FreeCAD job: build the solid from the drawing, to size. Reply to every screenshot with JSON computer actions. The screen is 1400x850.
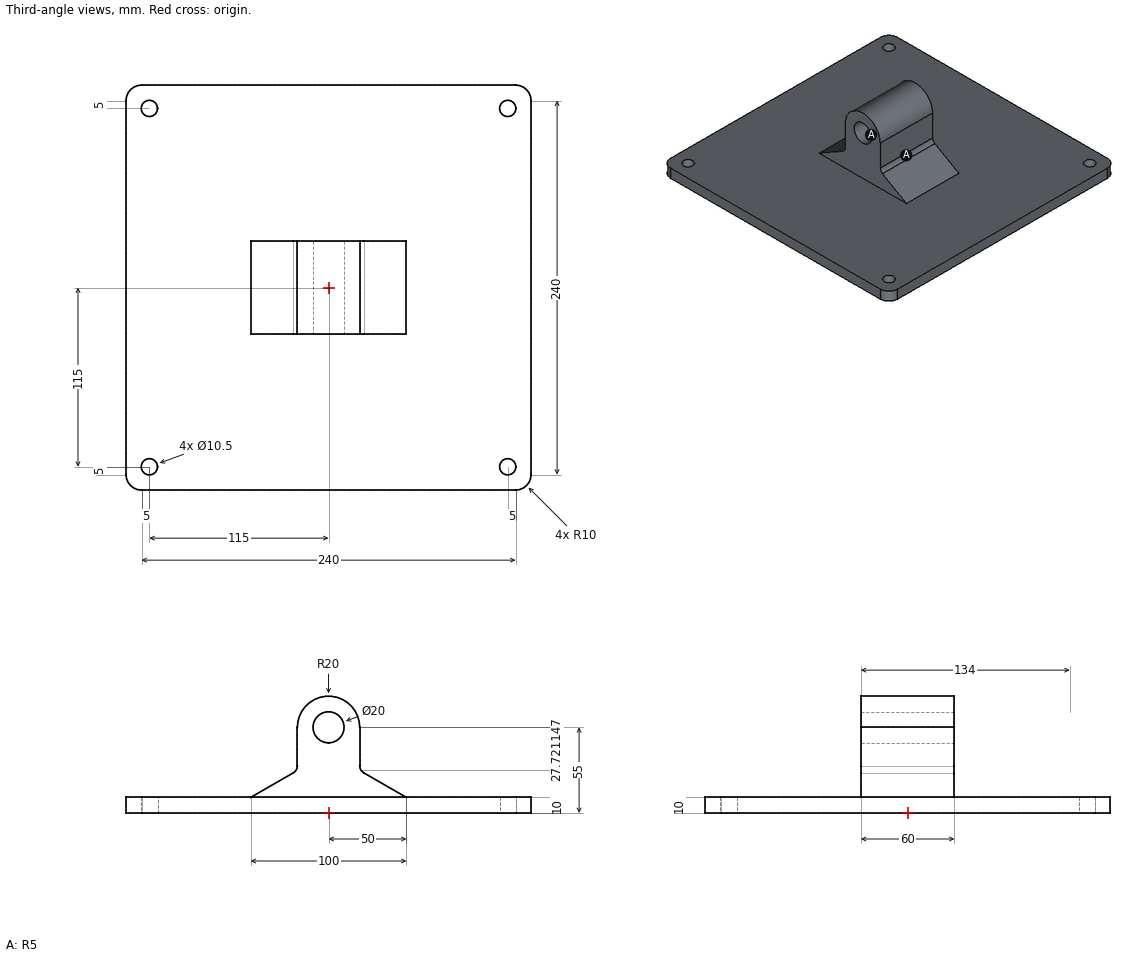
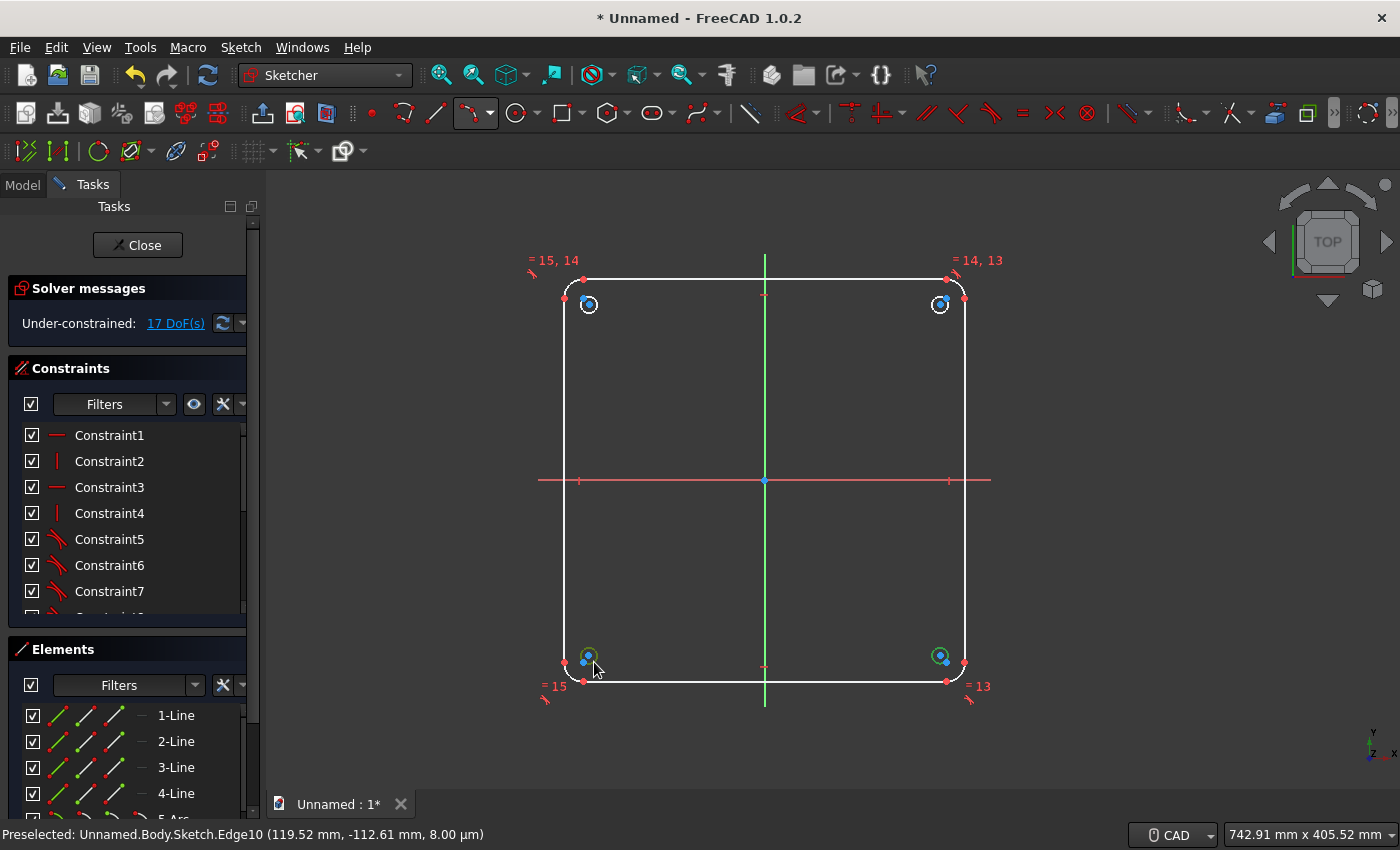
{"action": "scroll", "coordinate": [595, 299], "scroll_direction": "up", "scroll_amount": 3}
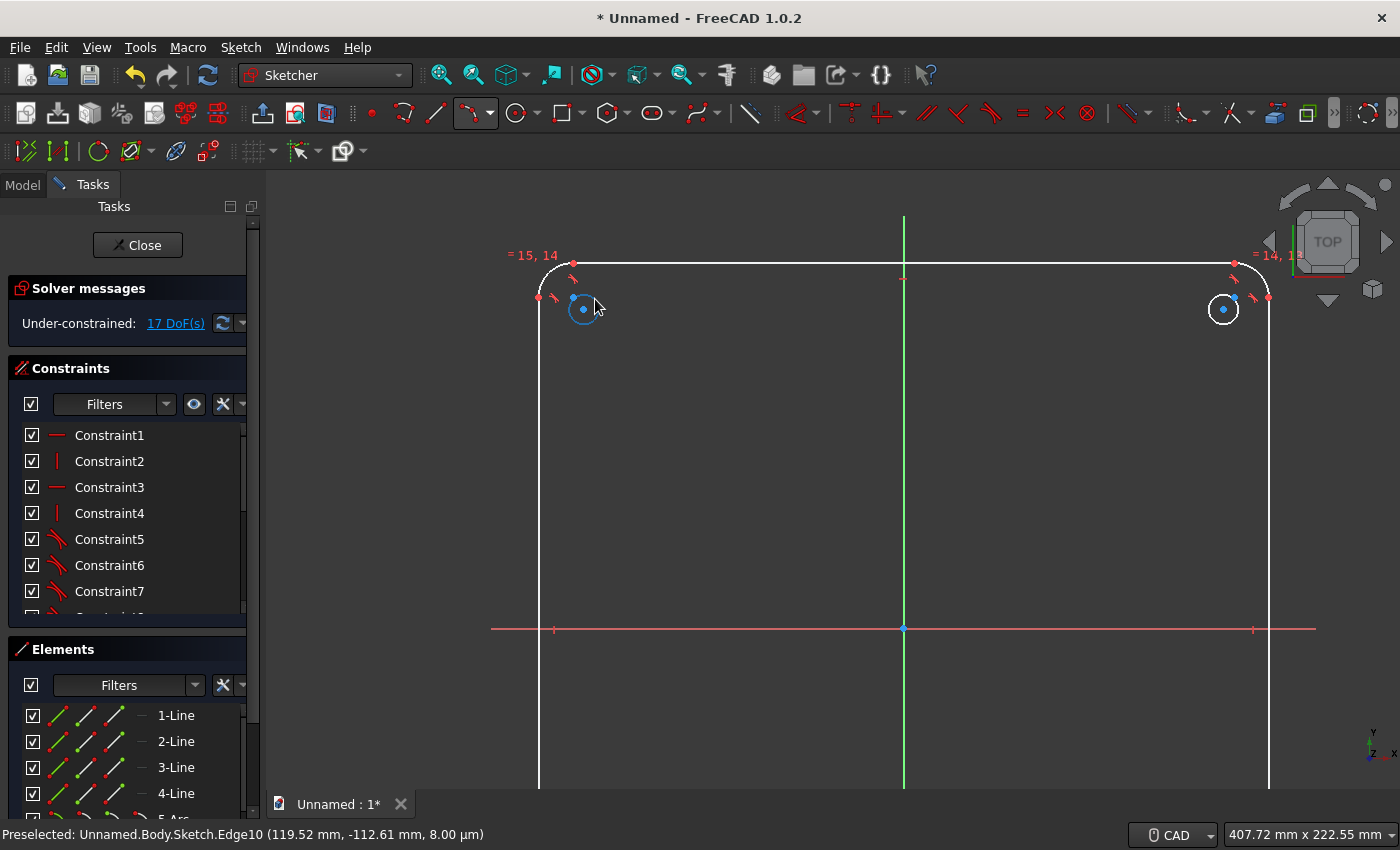
{"action": "left_click", "coordinate": [594, 299]}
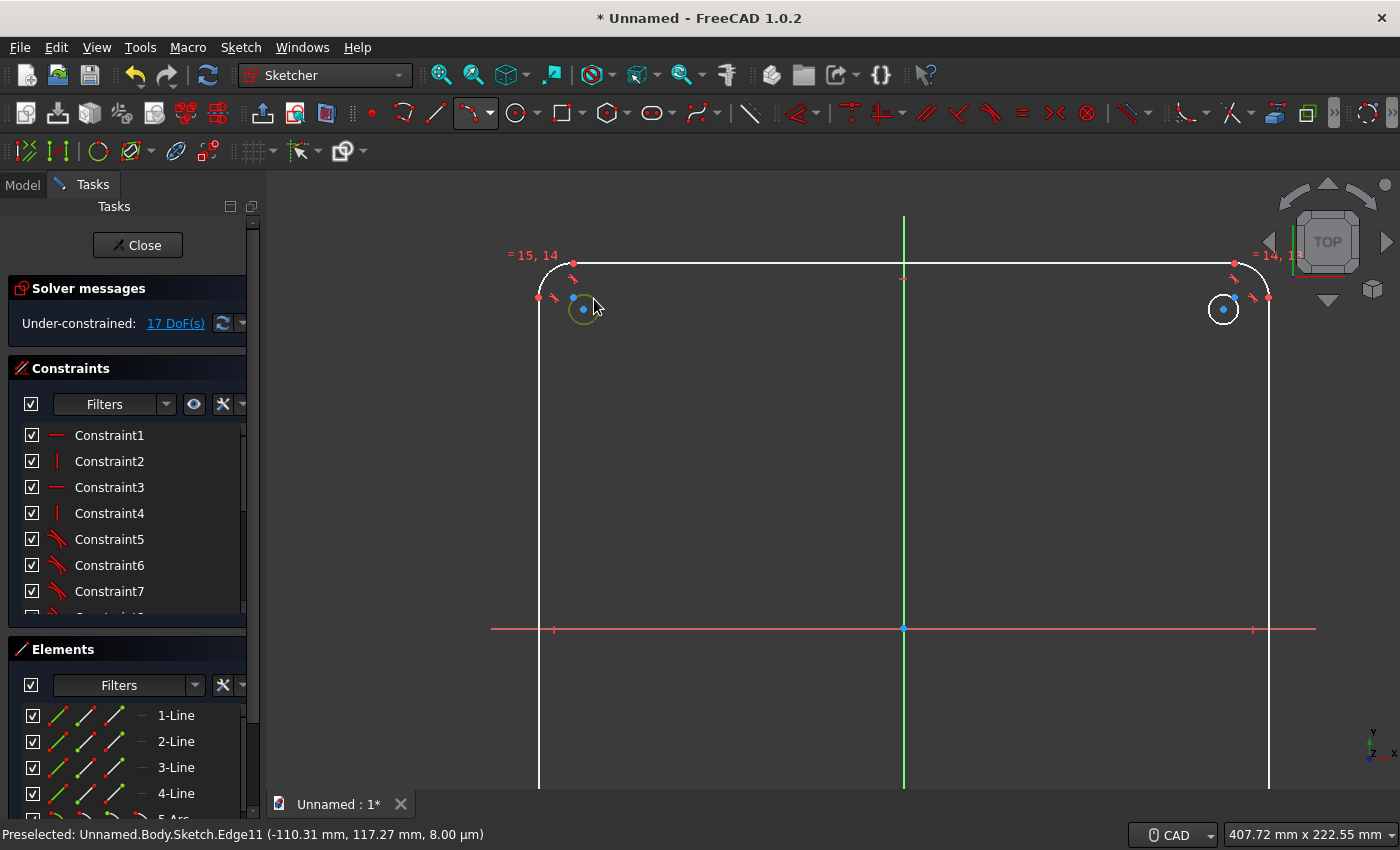
{"action": "left_click", "coordinate": [1213, 299]}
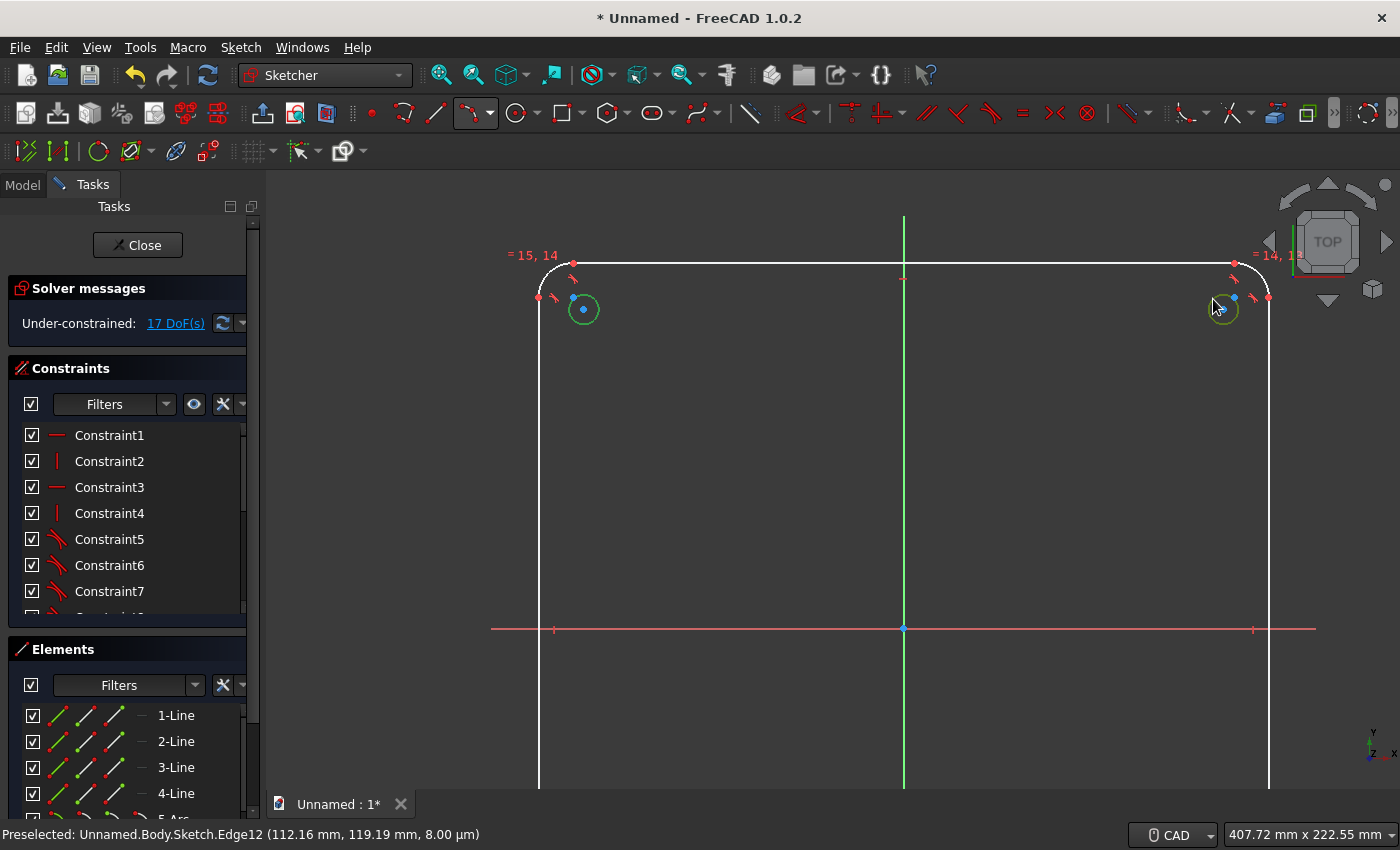
{"action": "left_click", "coordinate": [1024, 114]}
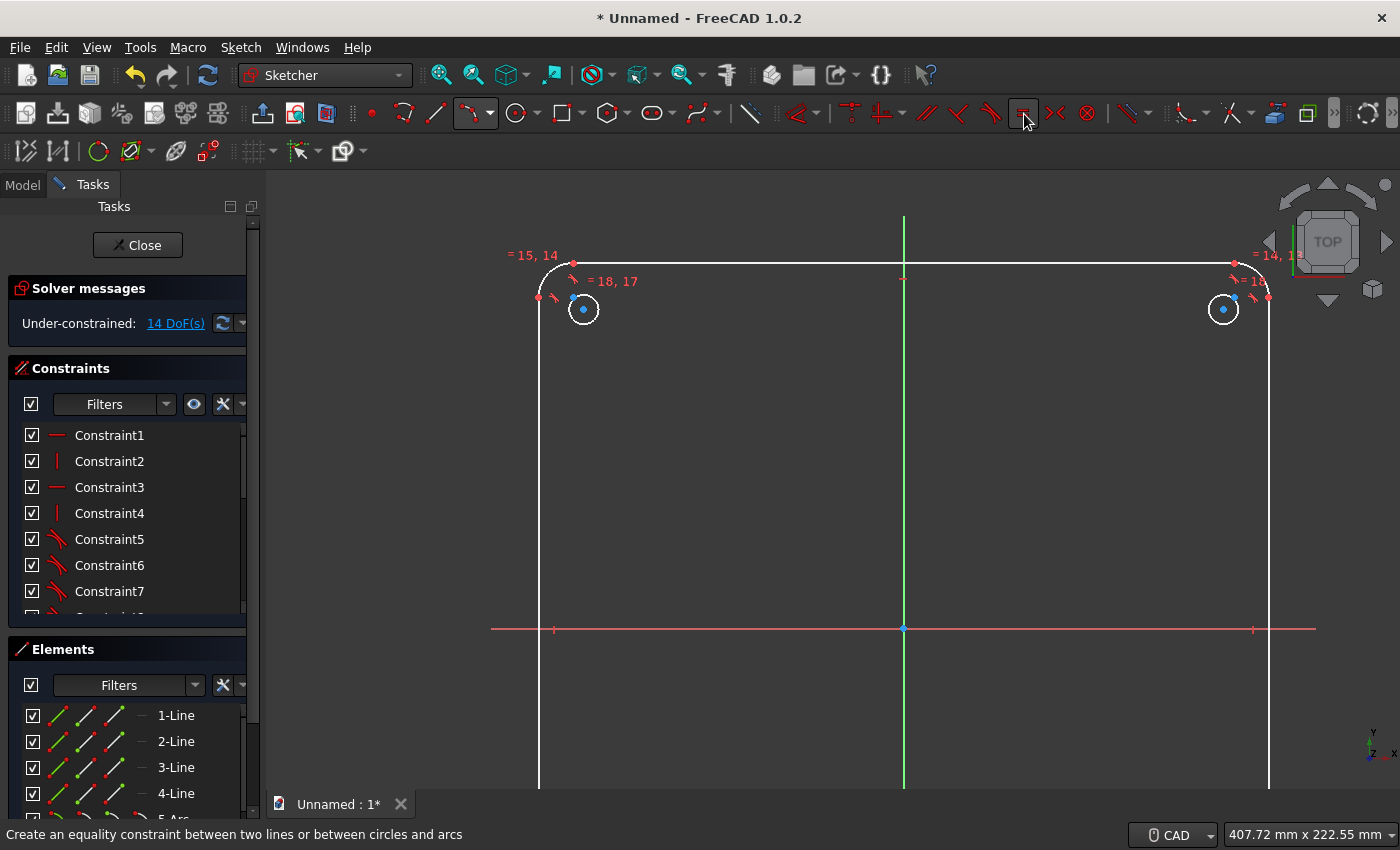
{"action": "scroll", "coordinate": [595, 298], "scroll_direction": "down", "scroll_amount": 3}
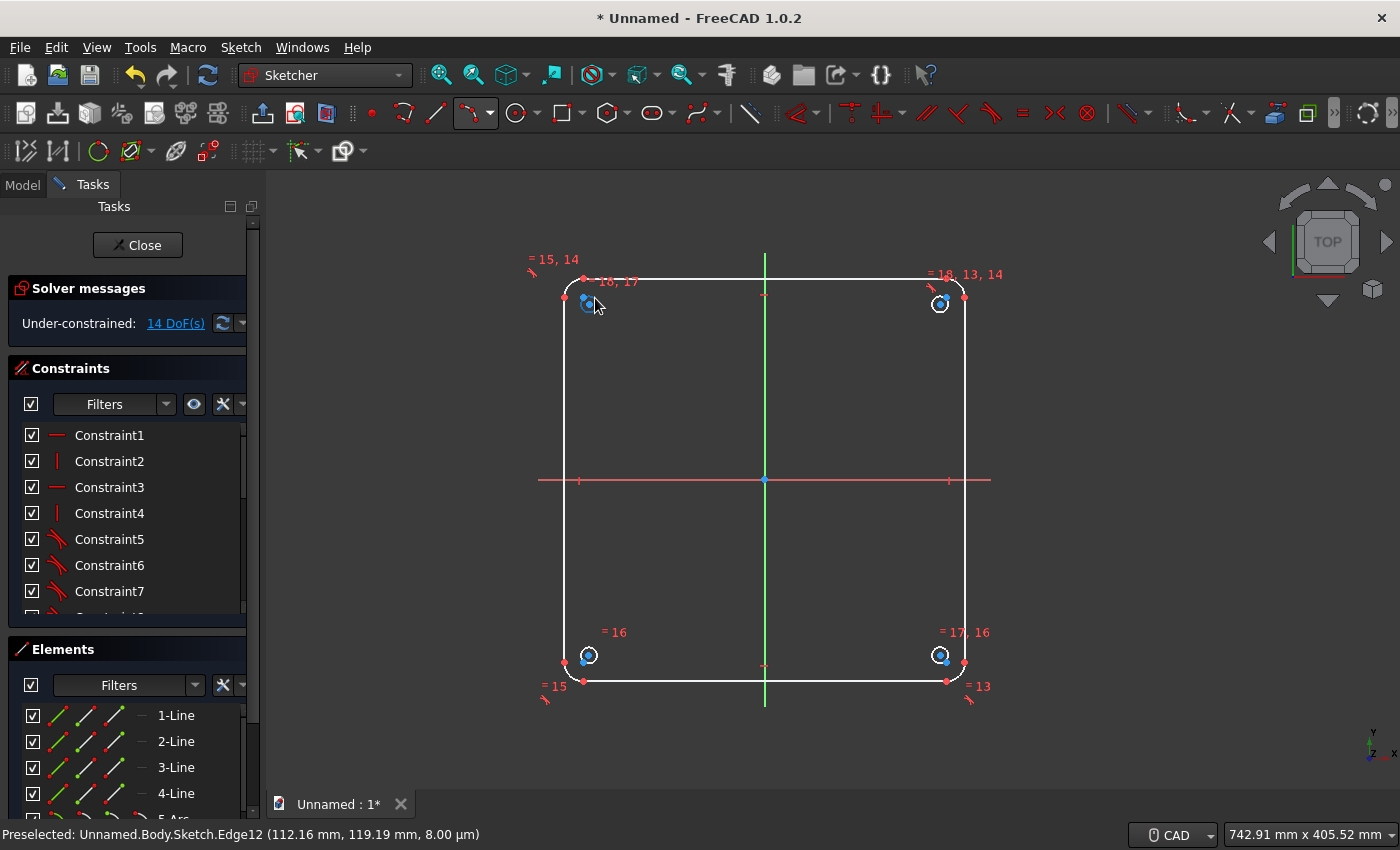
{"action": "scroll", "coordinate": [589, 655], "scroll_direction": "up", "scroll_amount": 2}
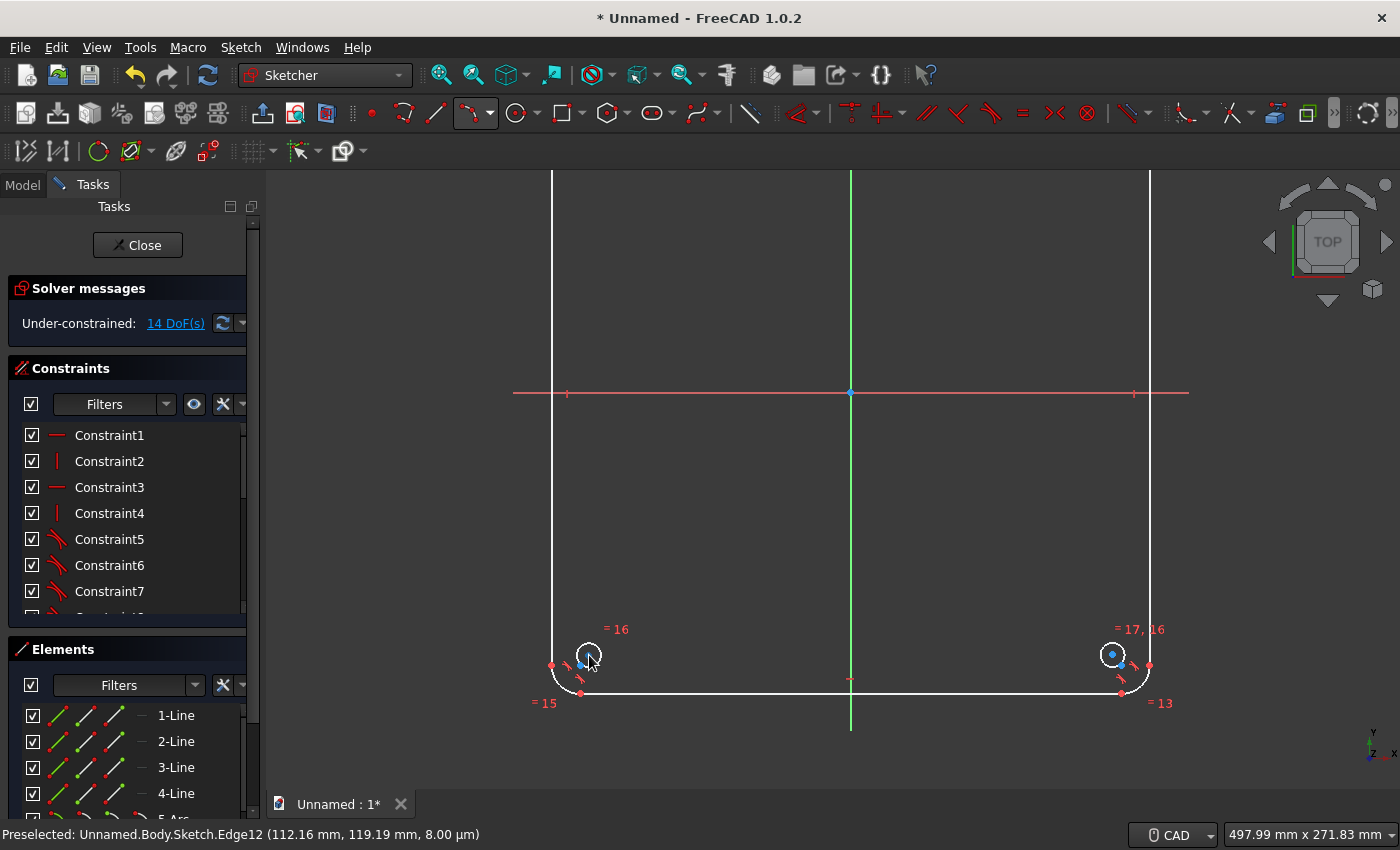
{"action": "left_click", "coordinate": [589, 655]}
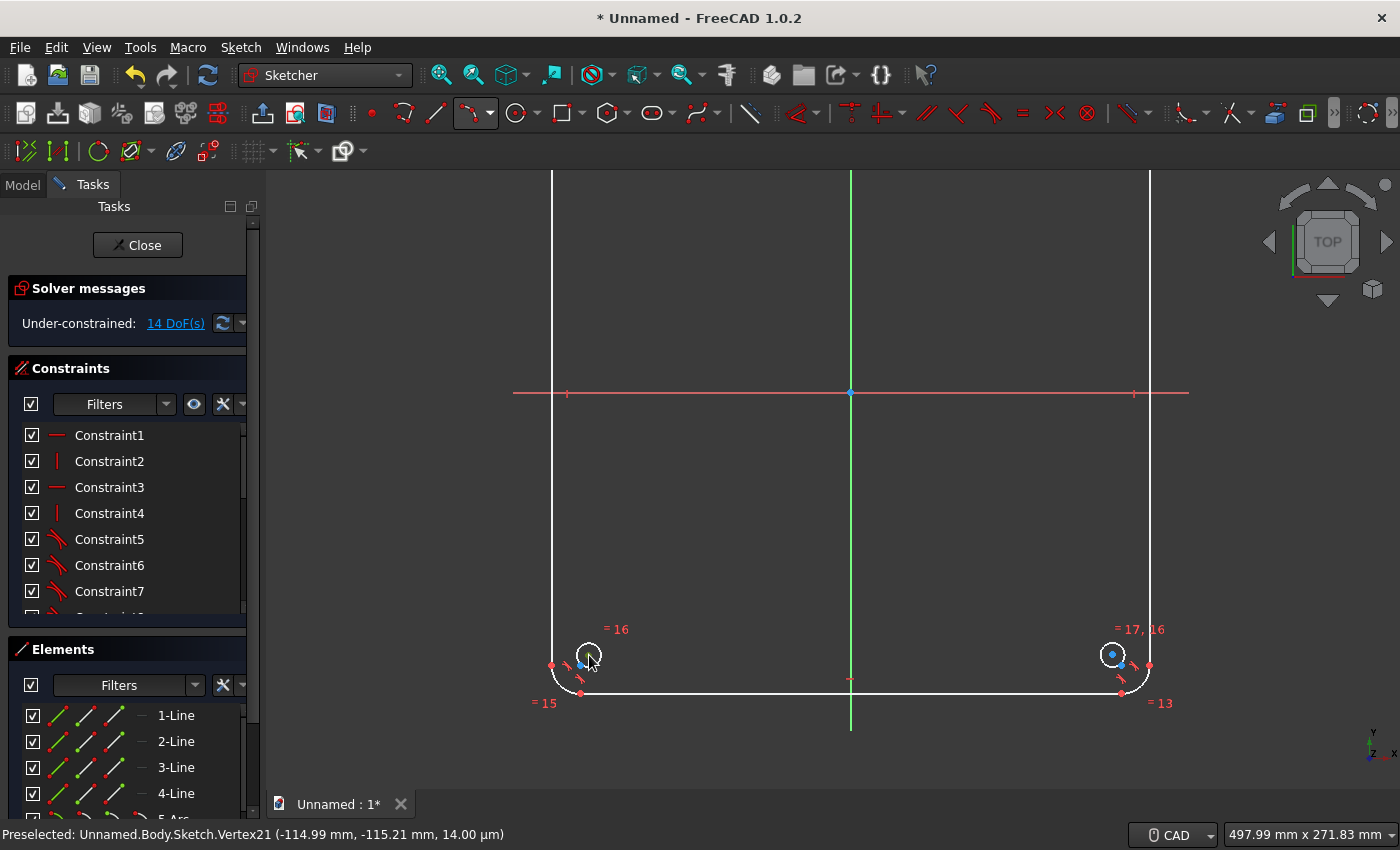
{"action": "left_click", "coordinate": [1113, 655]}